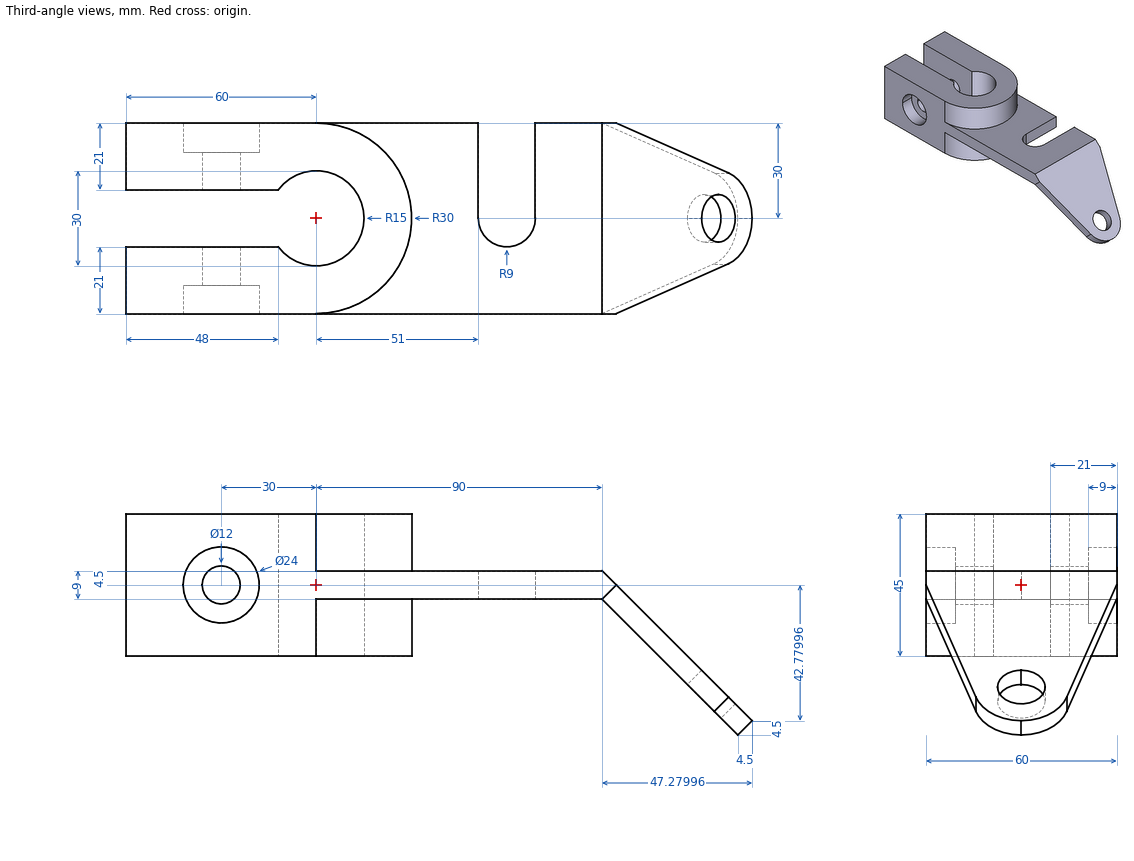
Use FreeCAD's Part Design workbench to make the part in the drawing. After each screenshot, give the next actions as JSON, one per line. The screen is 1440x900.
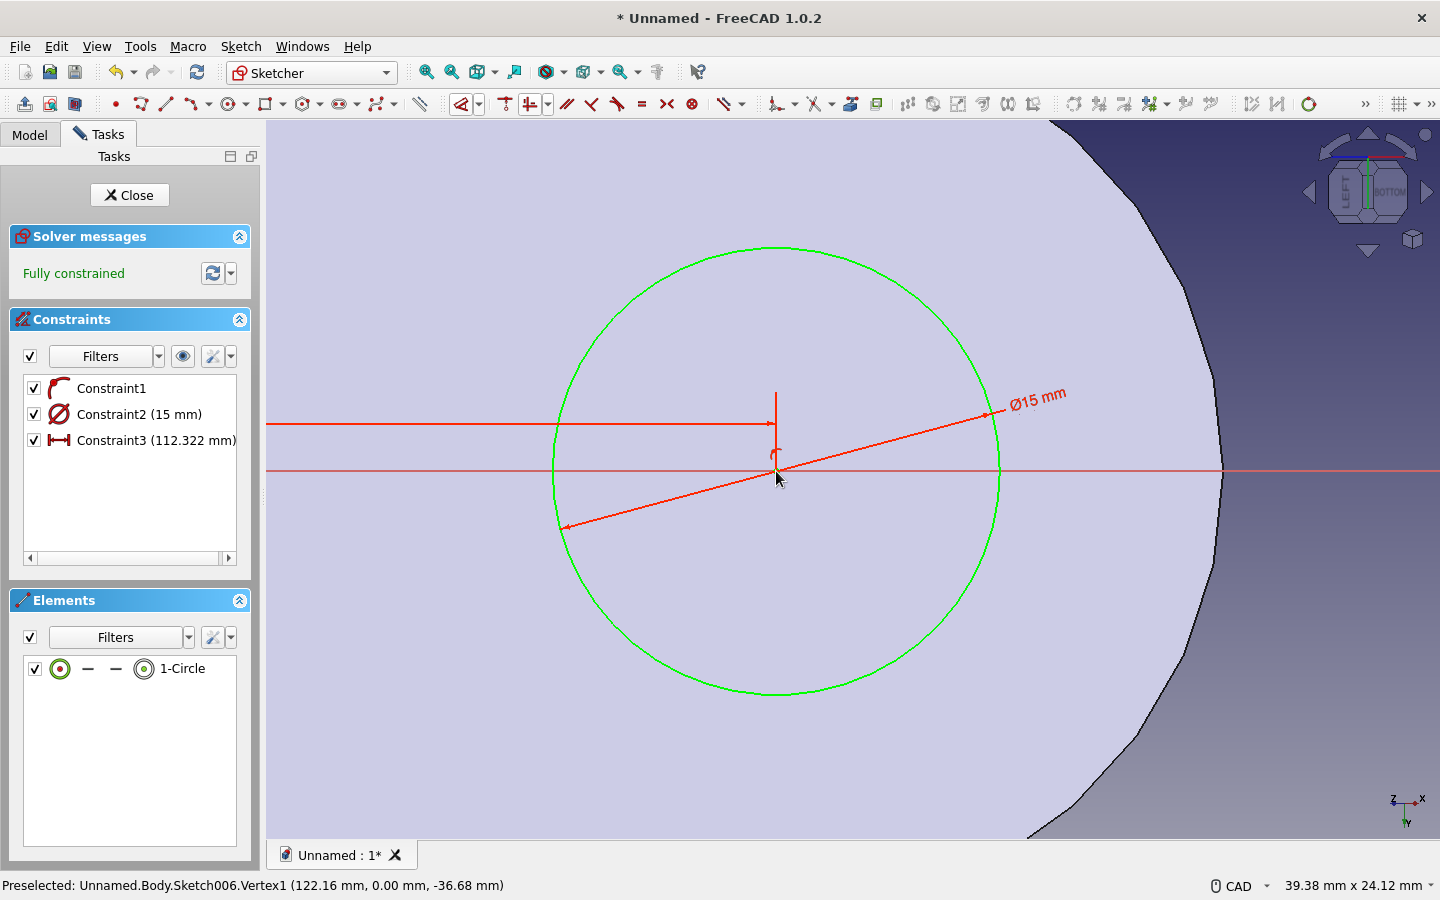
{"action": "left_click", "coordinate": [130, 195]}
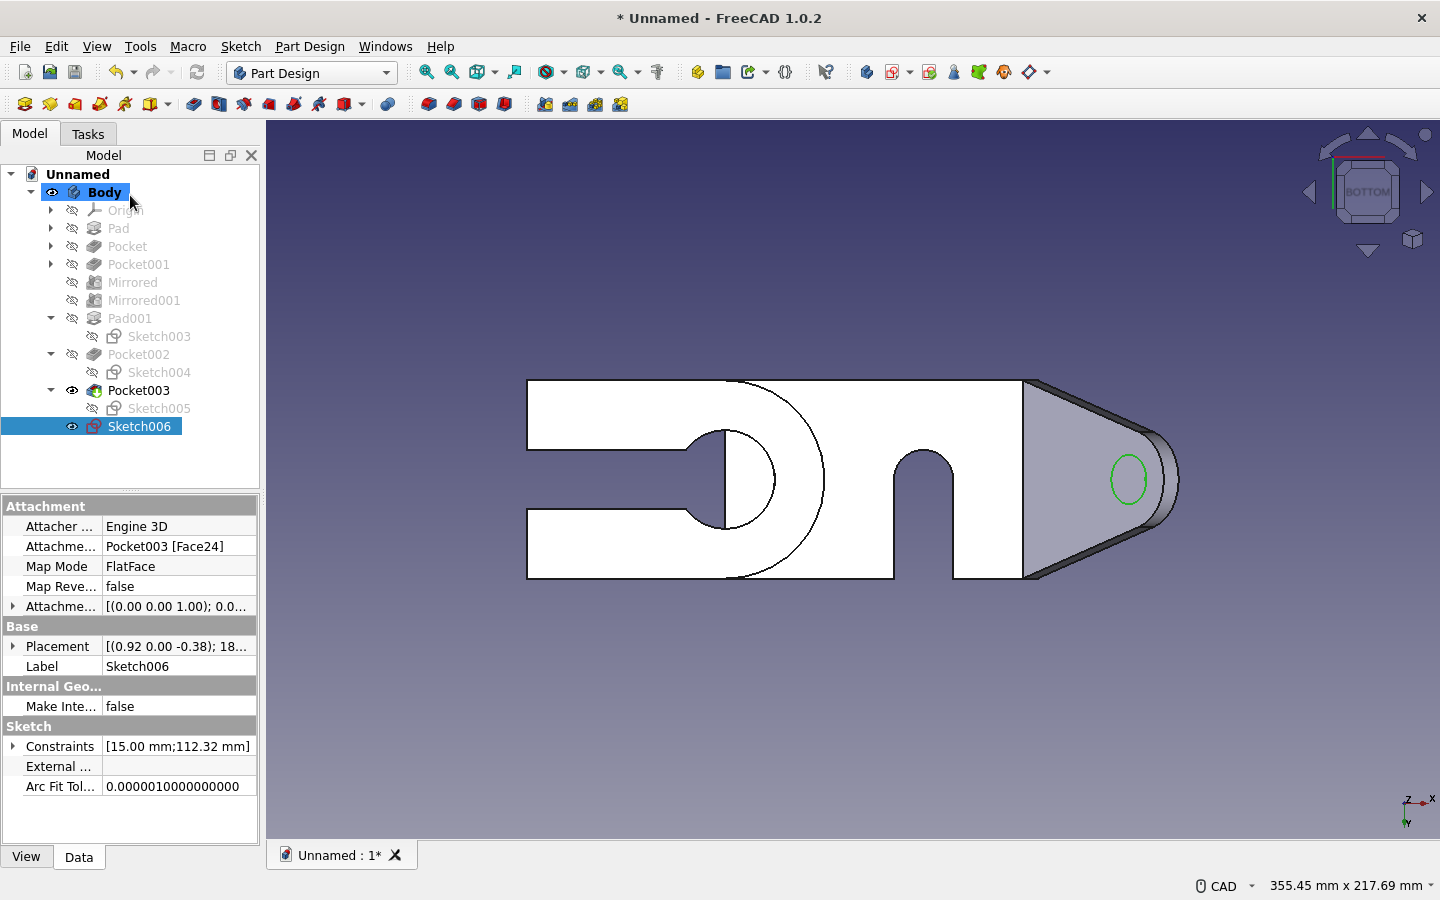
{"action": "left_click", "coordinate": [194, 104]}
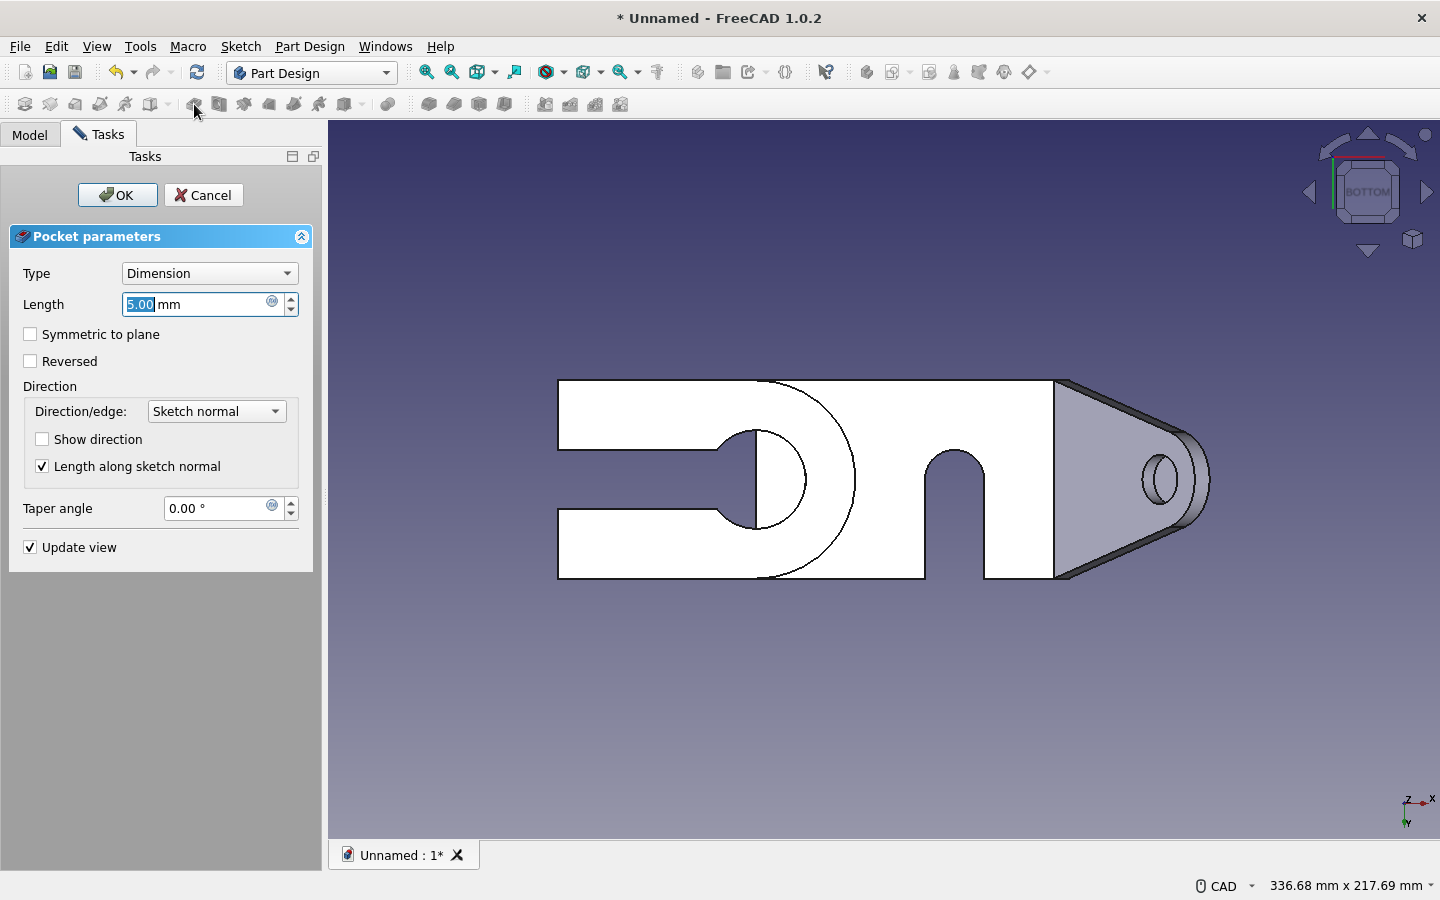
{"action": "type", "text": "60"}
{"action": "key", "text": "Tab"}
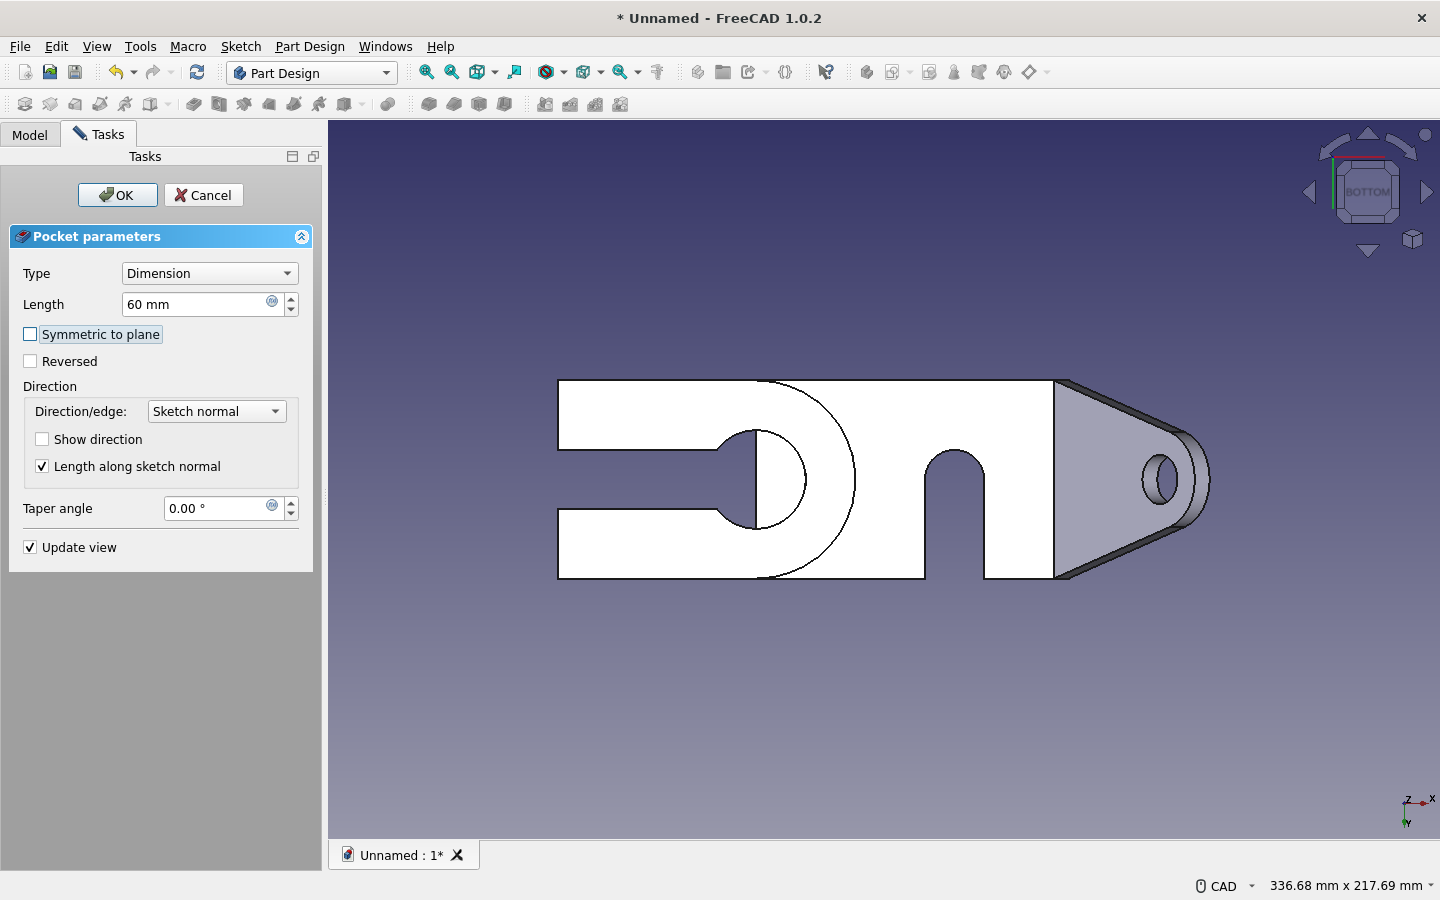
{"action": "left_click", "coordinate": [31, 334]}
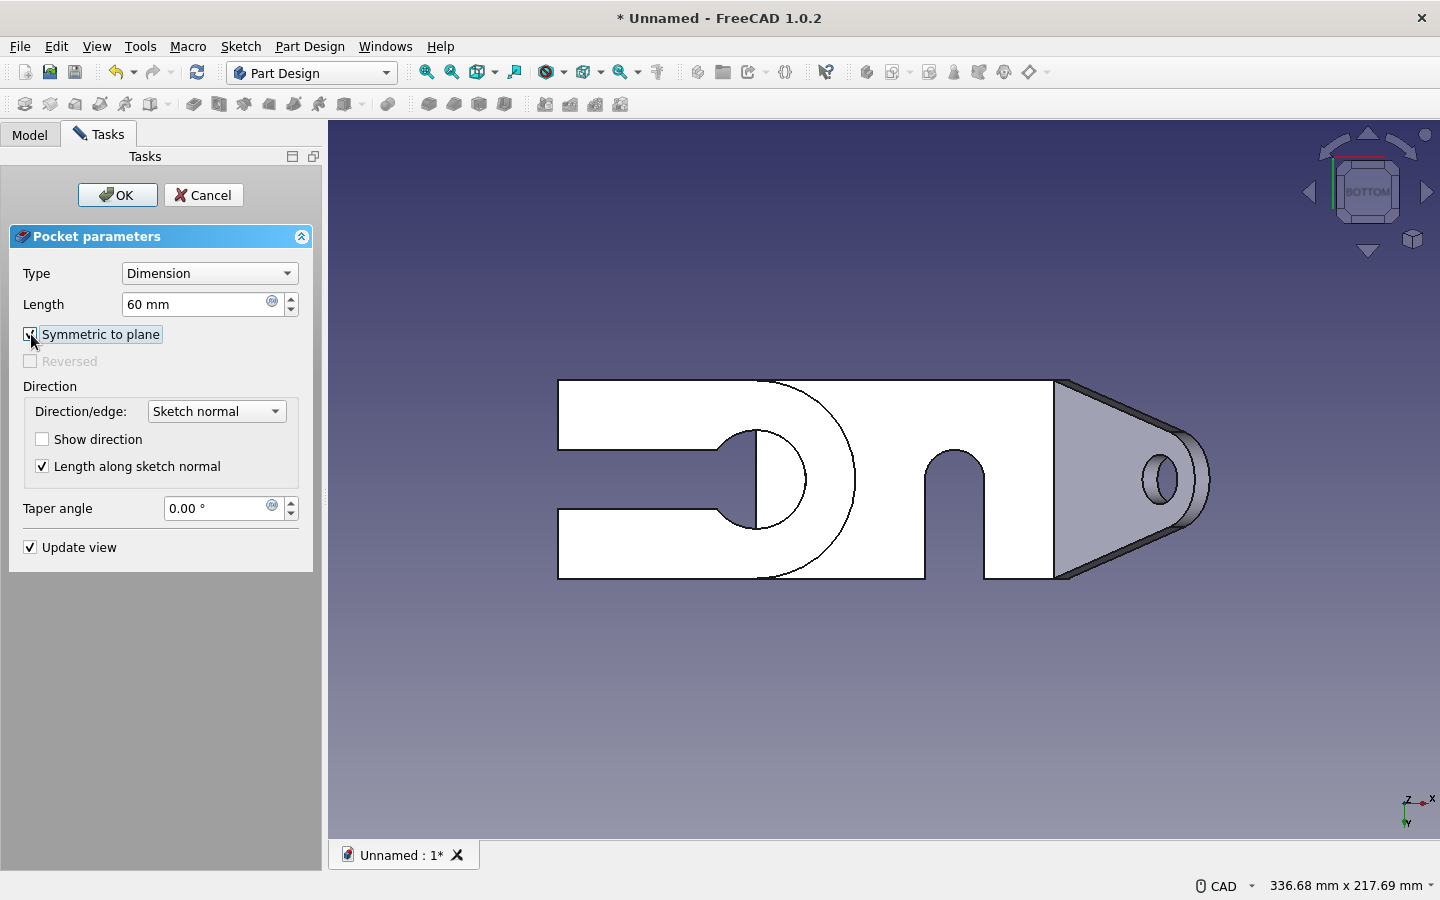
{"action": "left_click", "coordinate": [118, 195]}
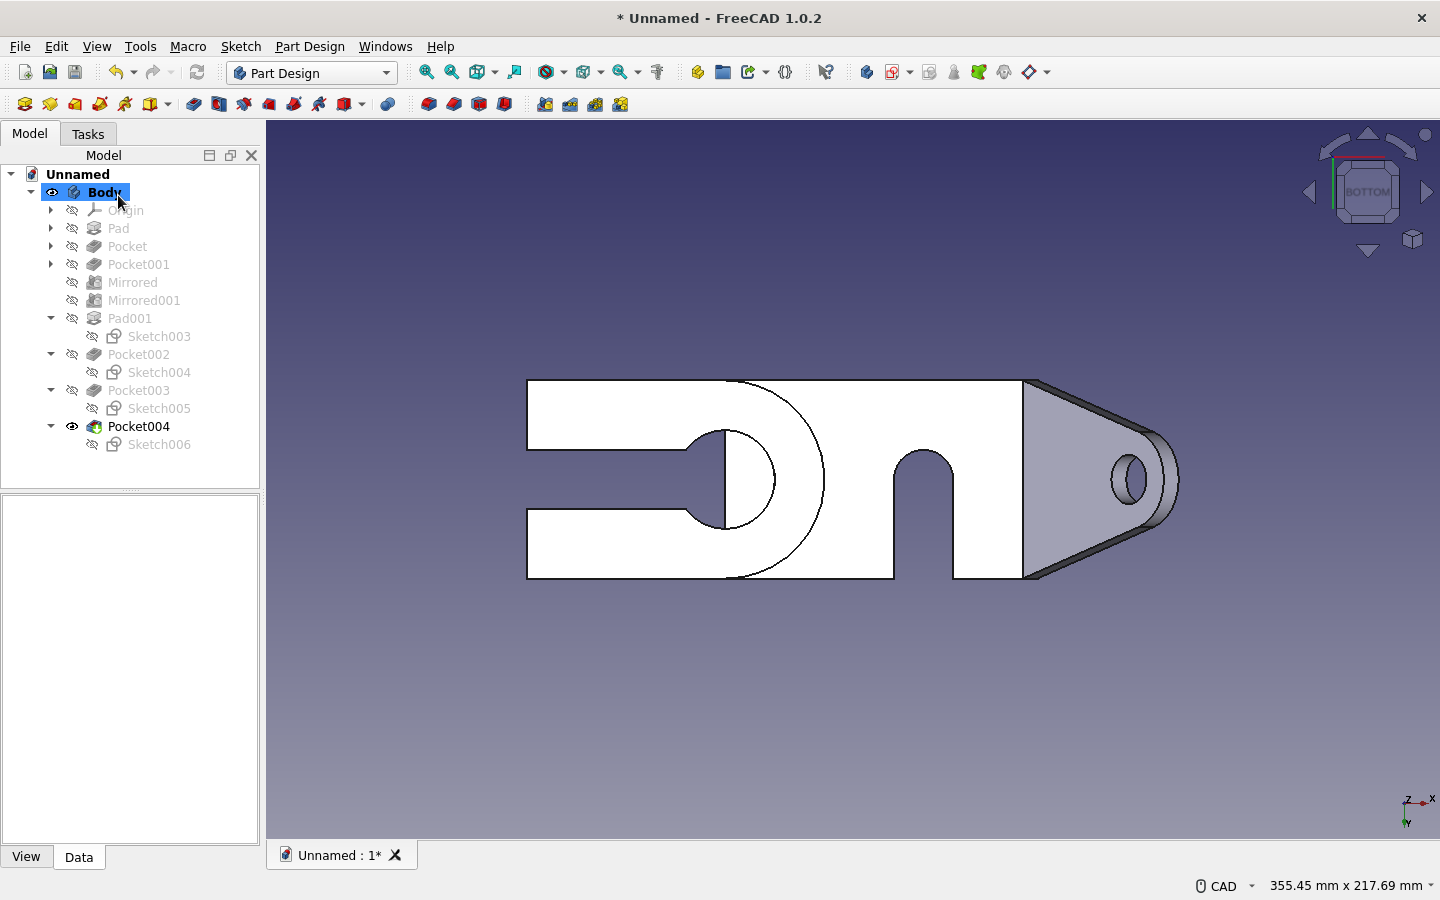
{"action": "left_click", "coordinate": [633, 422]}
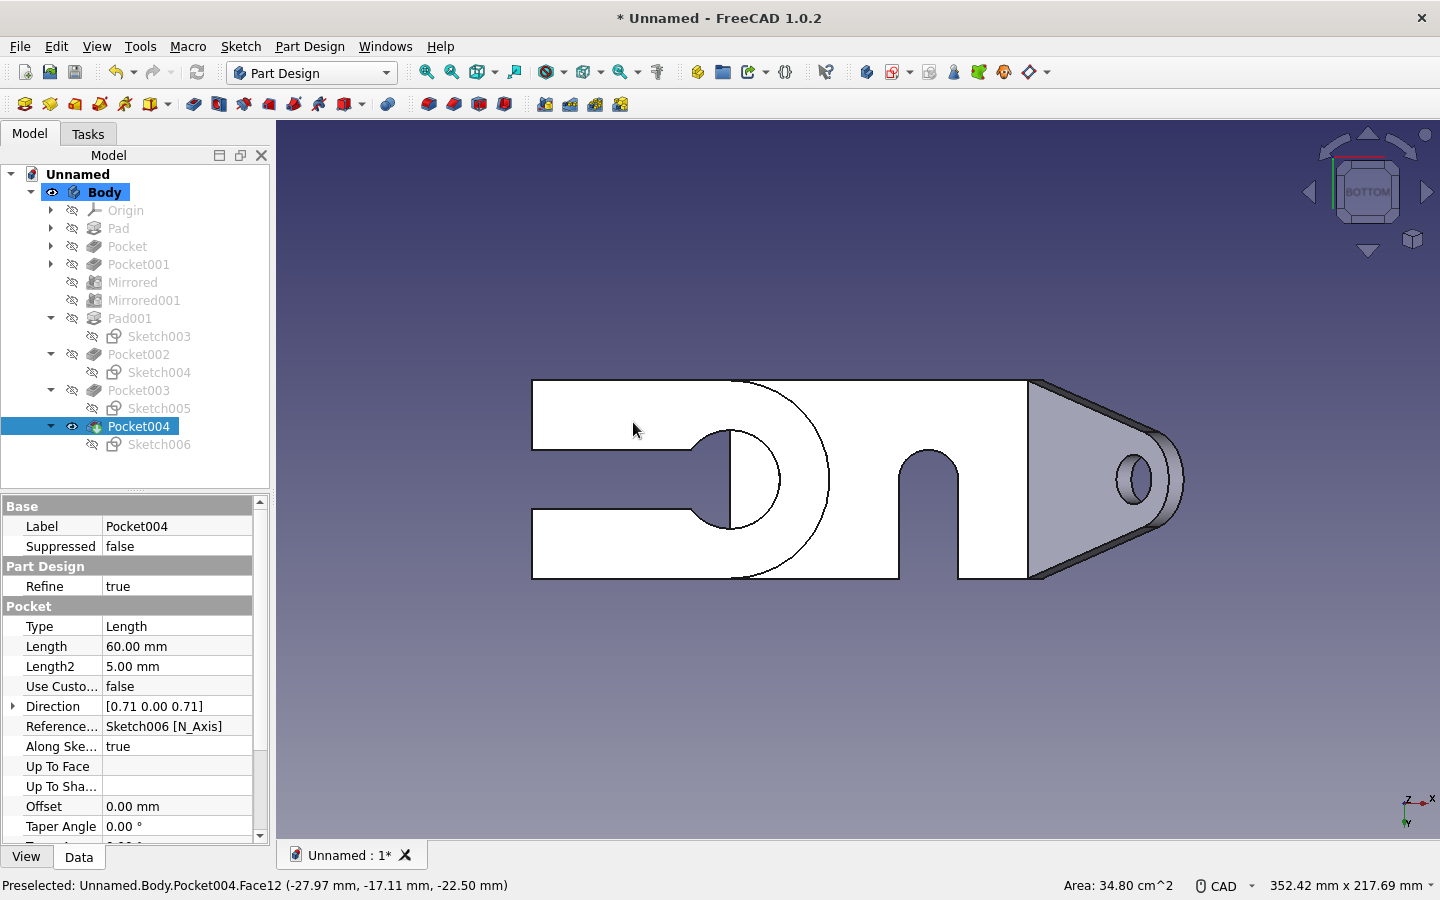
{"action": "left_click", "coordinate": [892, 72]}